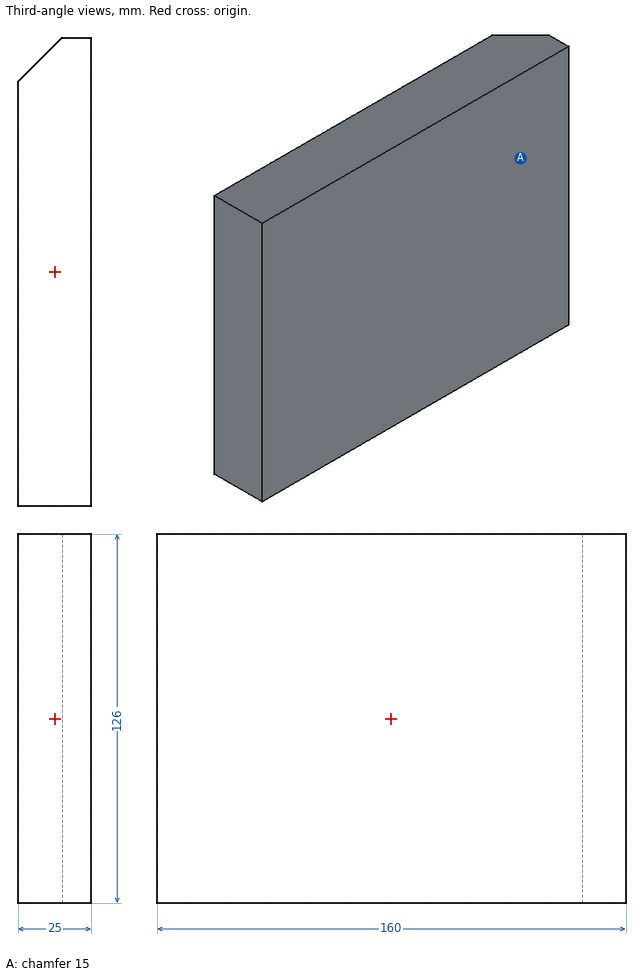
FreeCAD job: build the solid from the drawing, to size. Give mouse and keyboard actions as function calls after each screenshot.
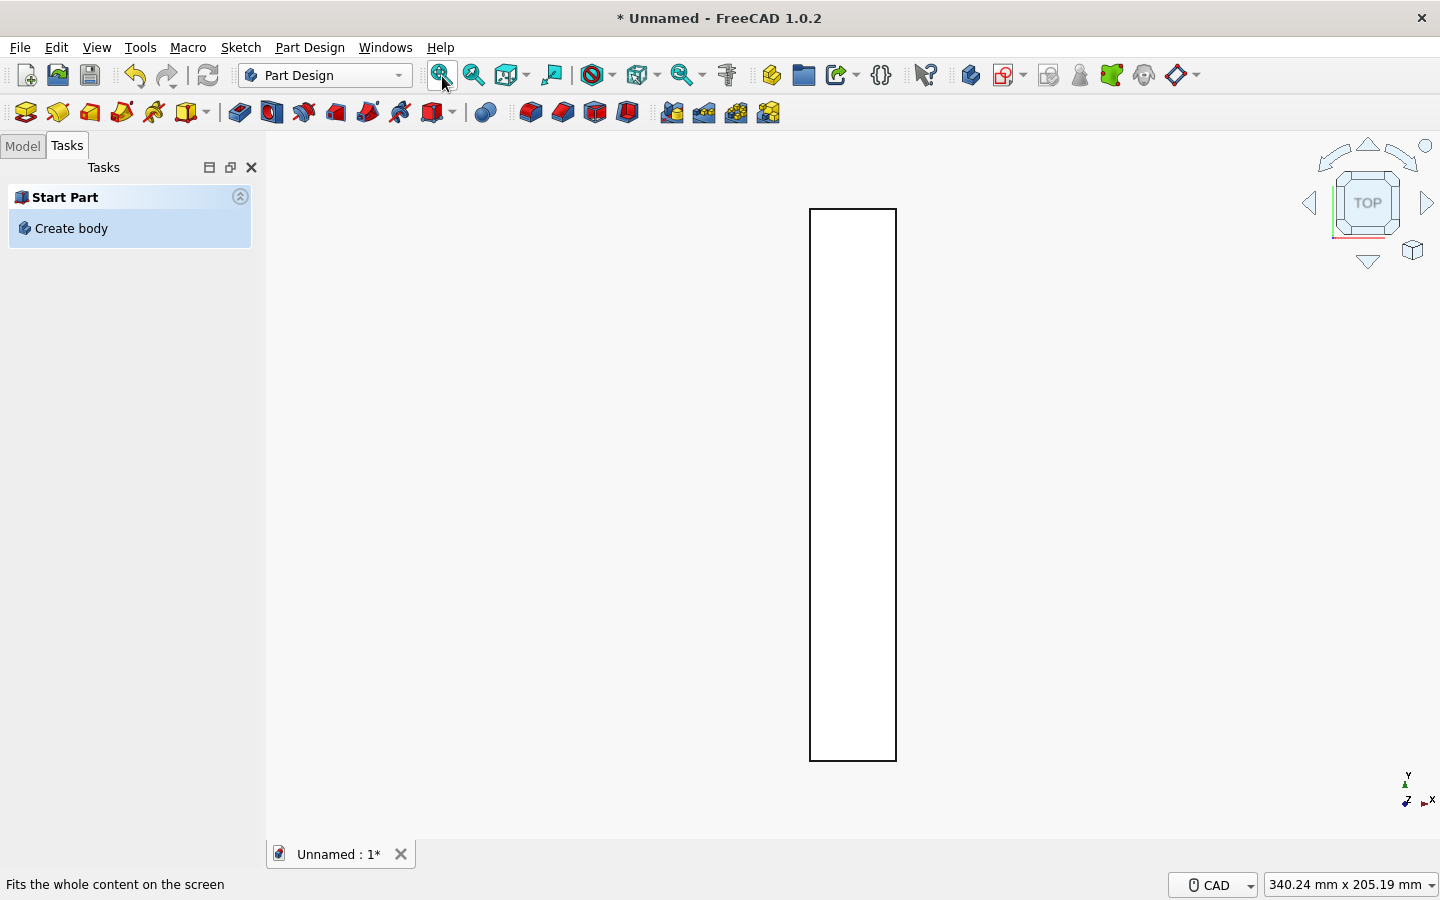
key(1)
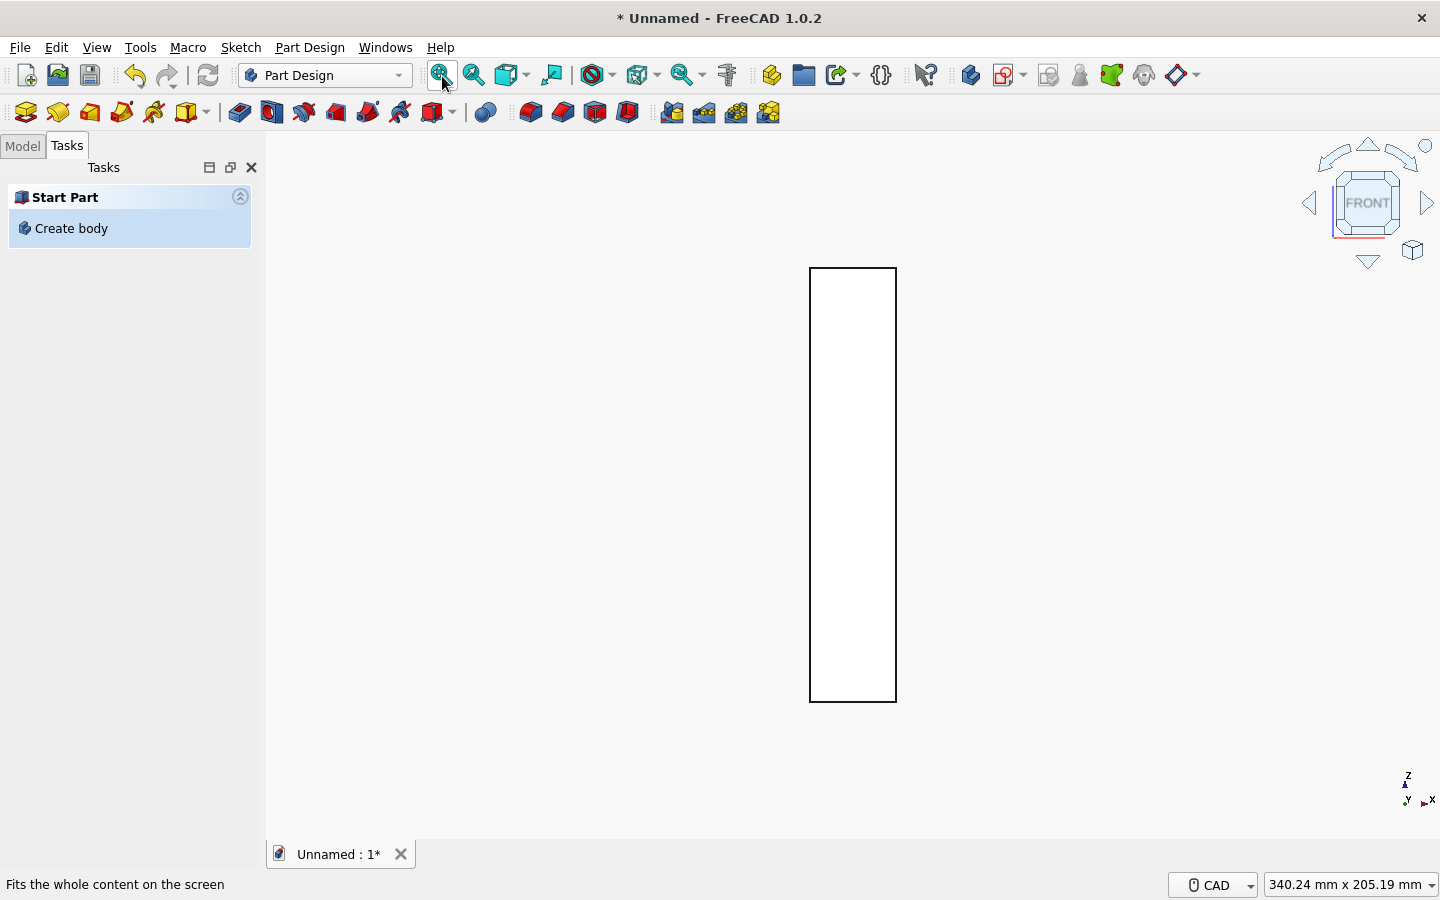
key(3)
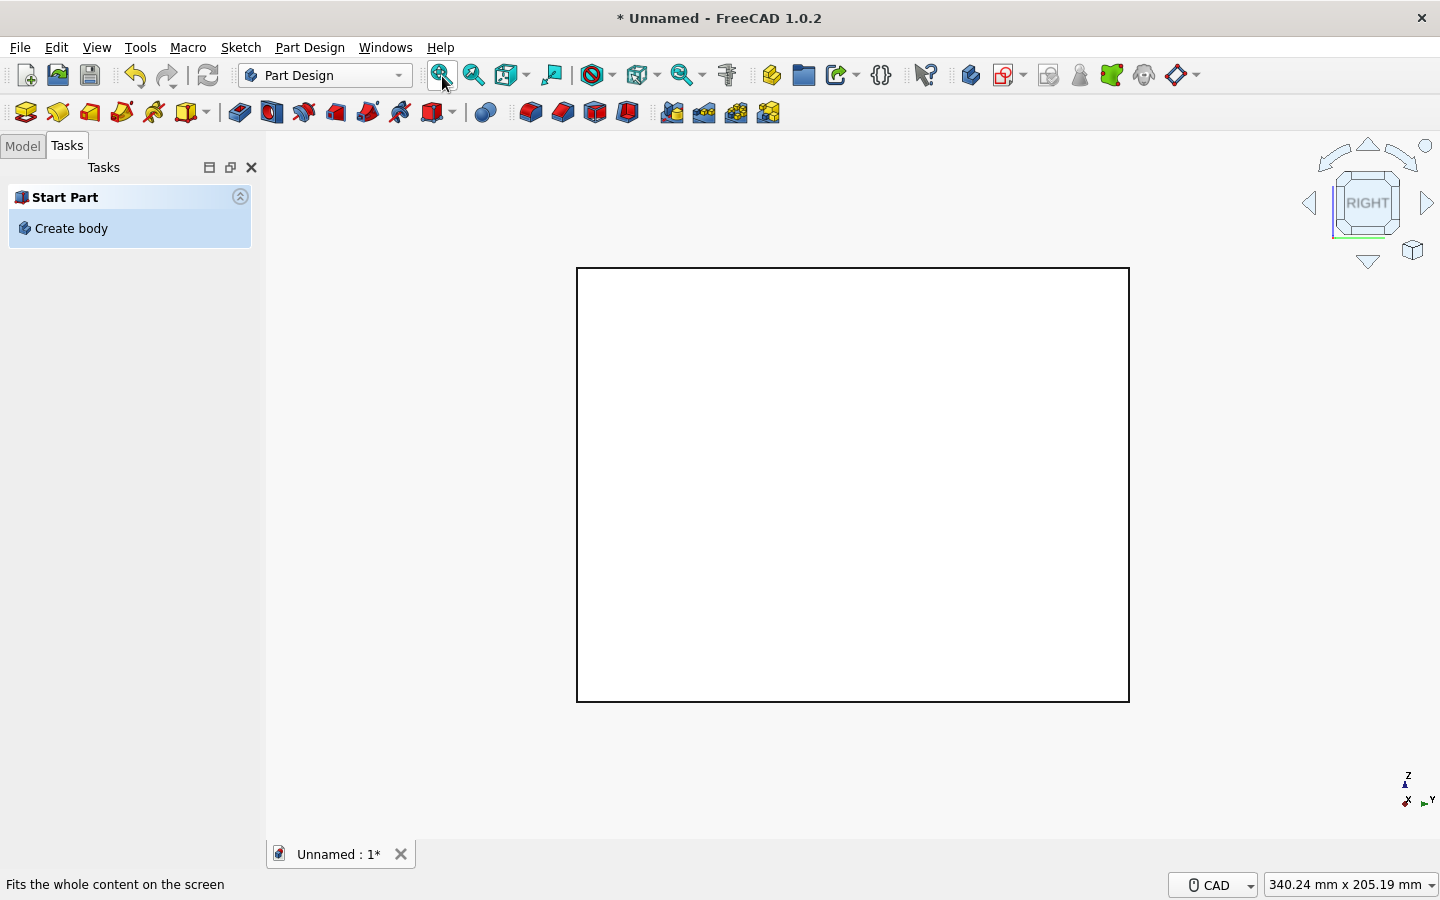
key(5)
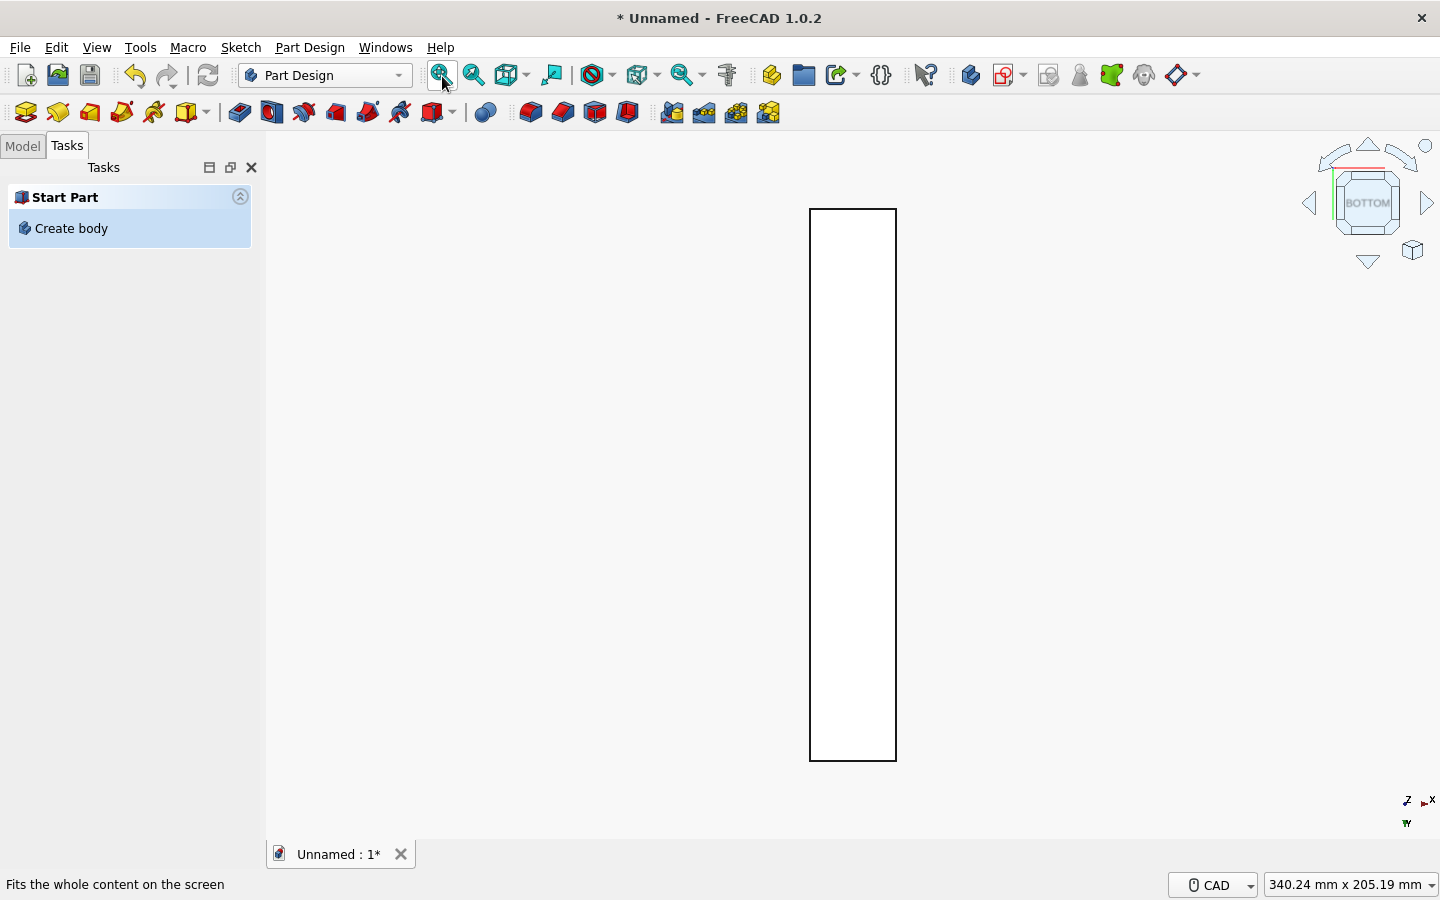
key(4)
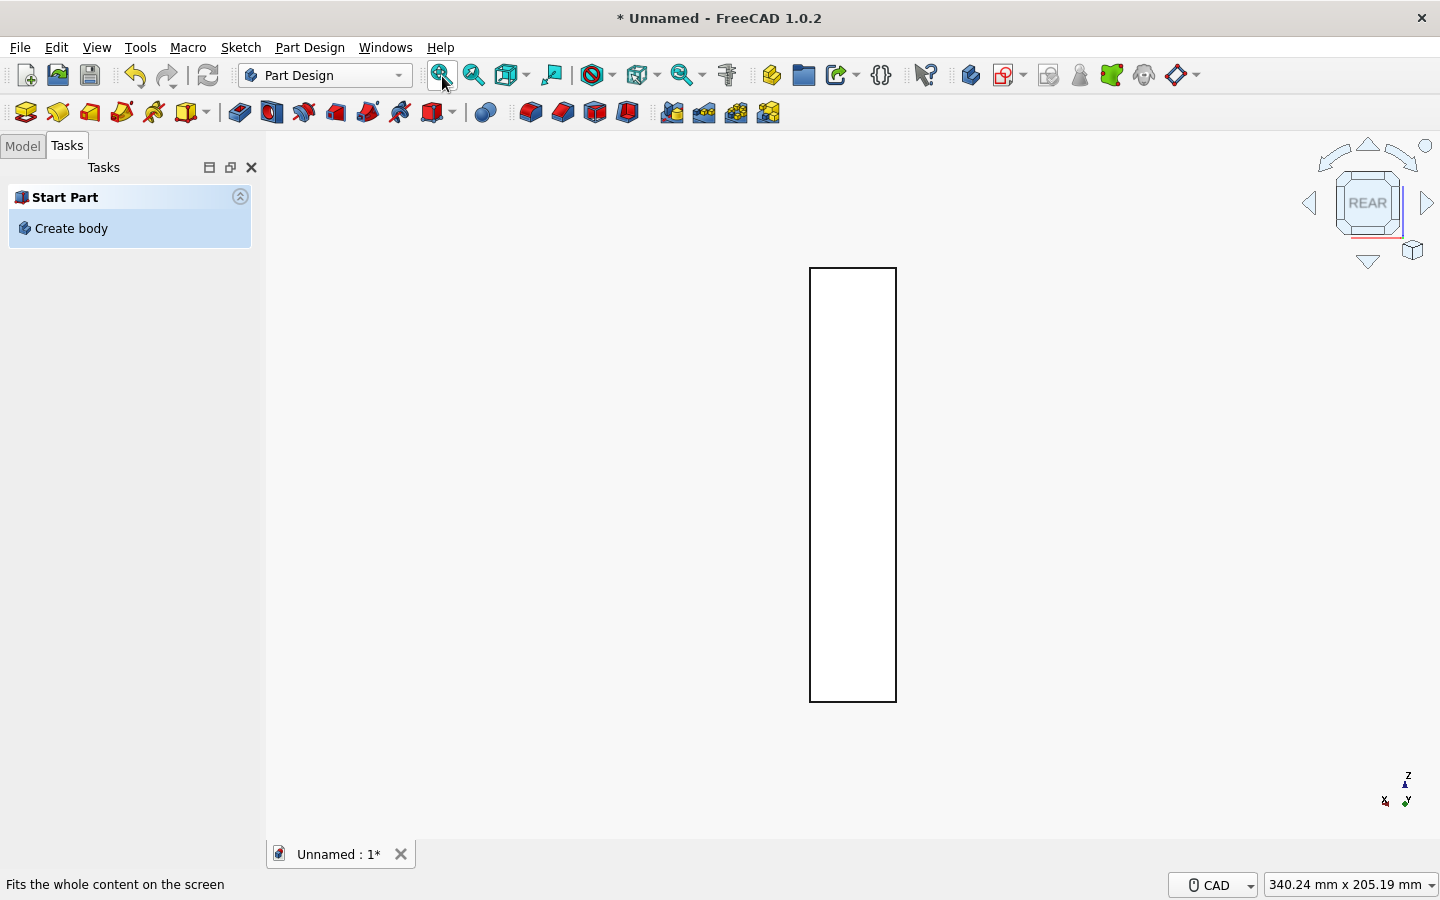
click(896, 484)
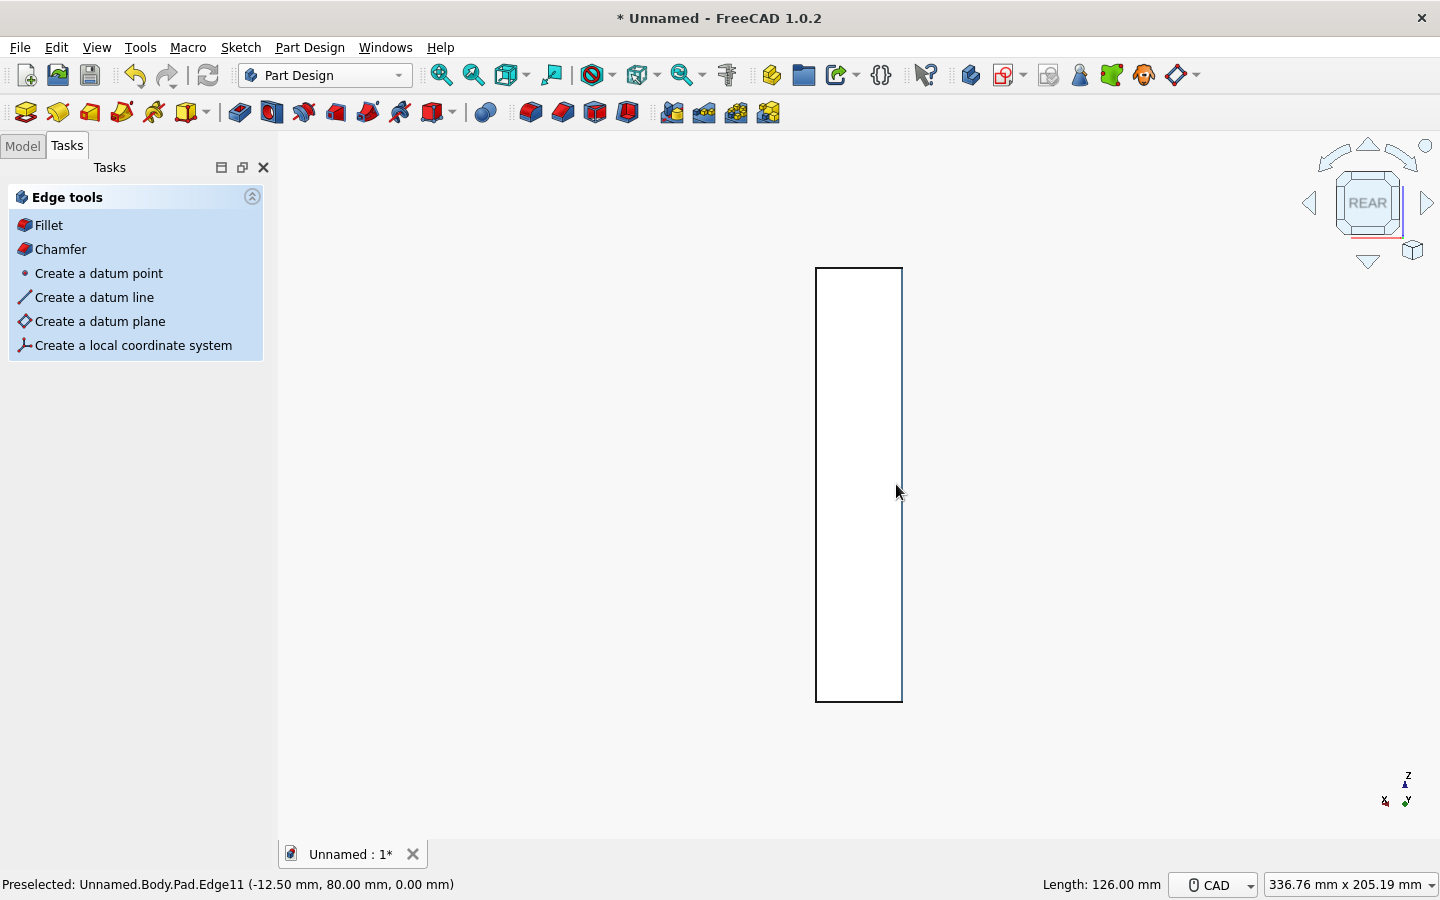
click(564, 112)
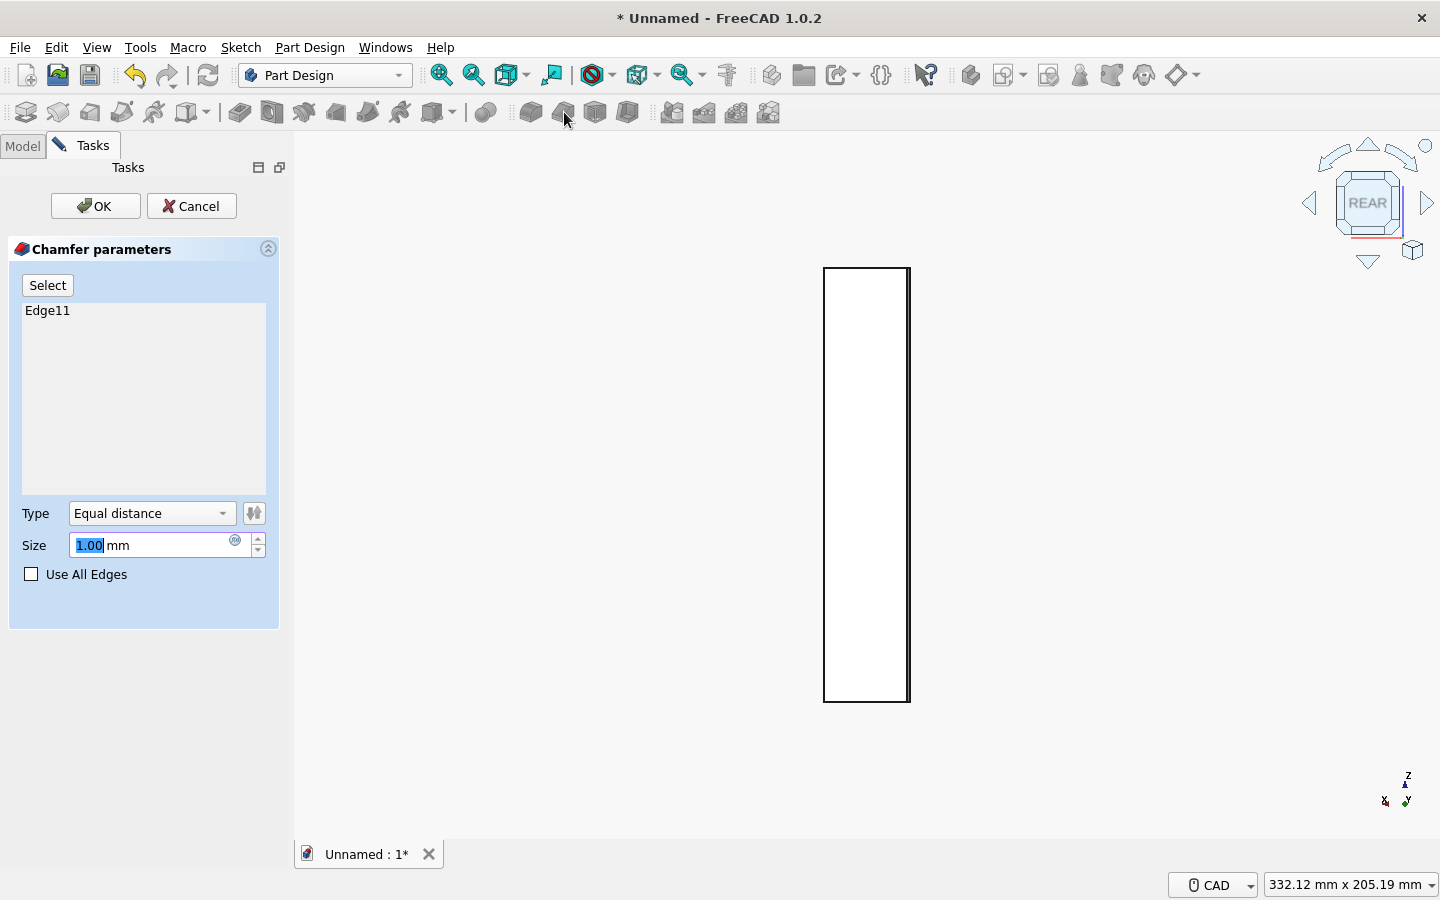
text(15)
key(Tab)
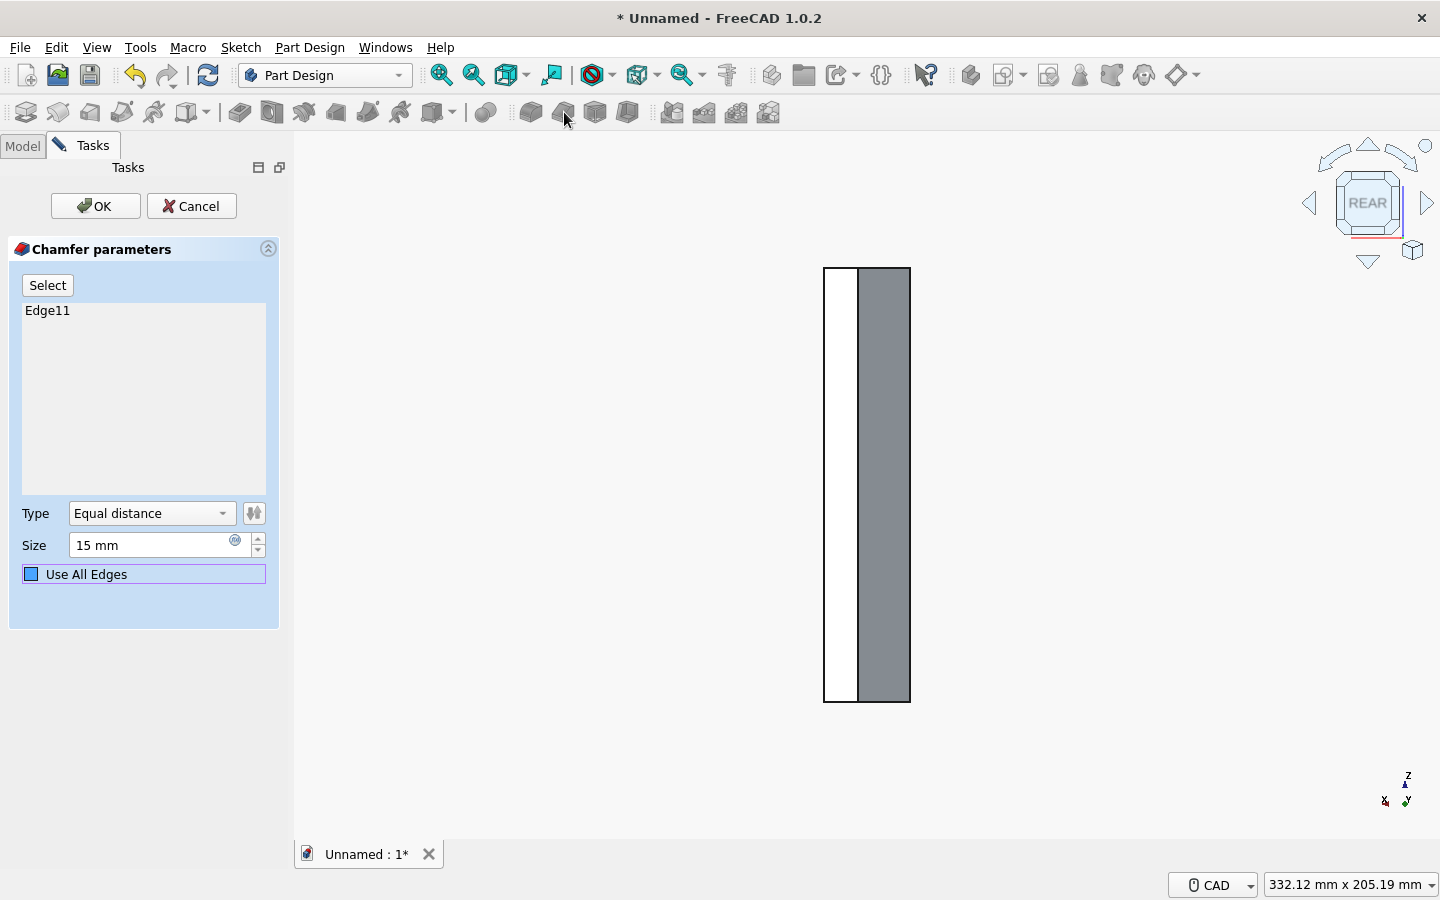
click(96, 206)